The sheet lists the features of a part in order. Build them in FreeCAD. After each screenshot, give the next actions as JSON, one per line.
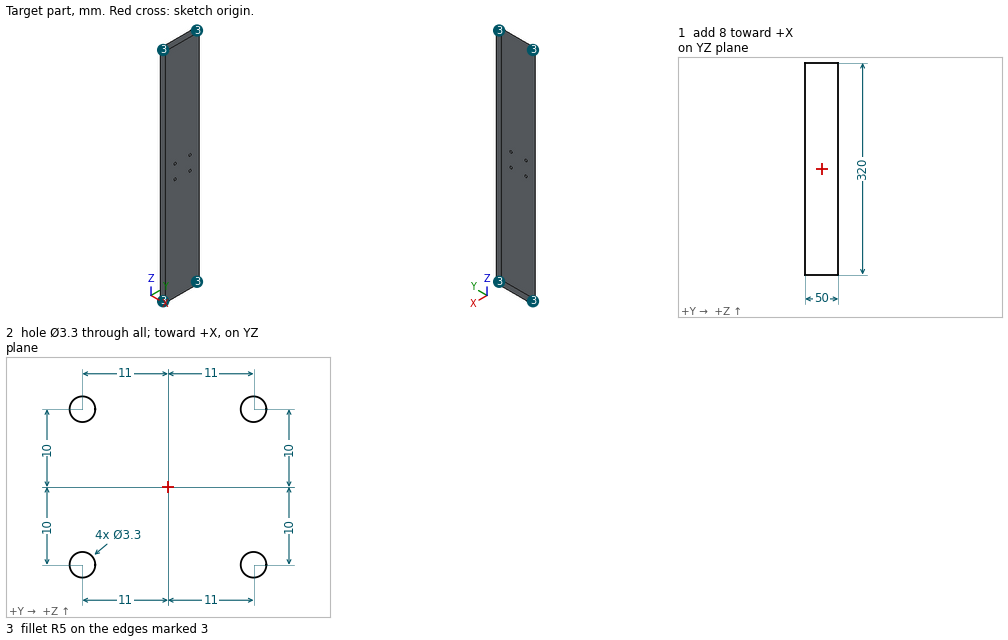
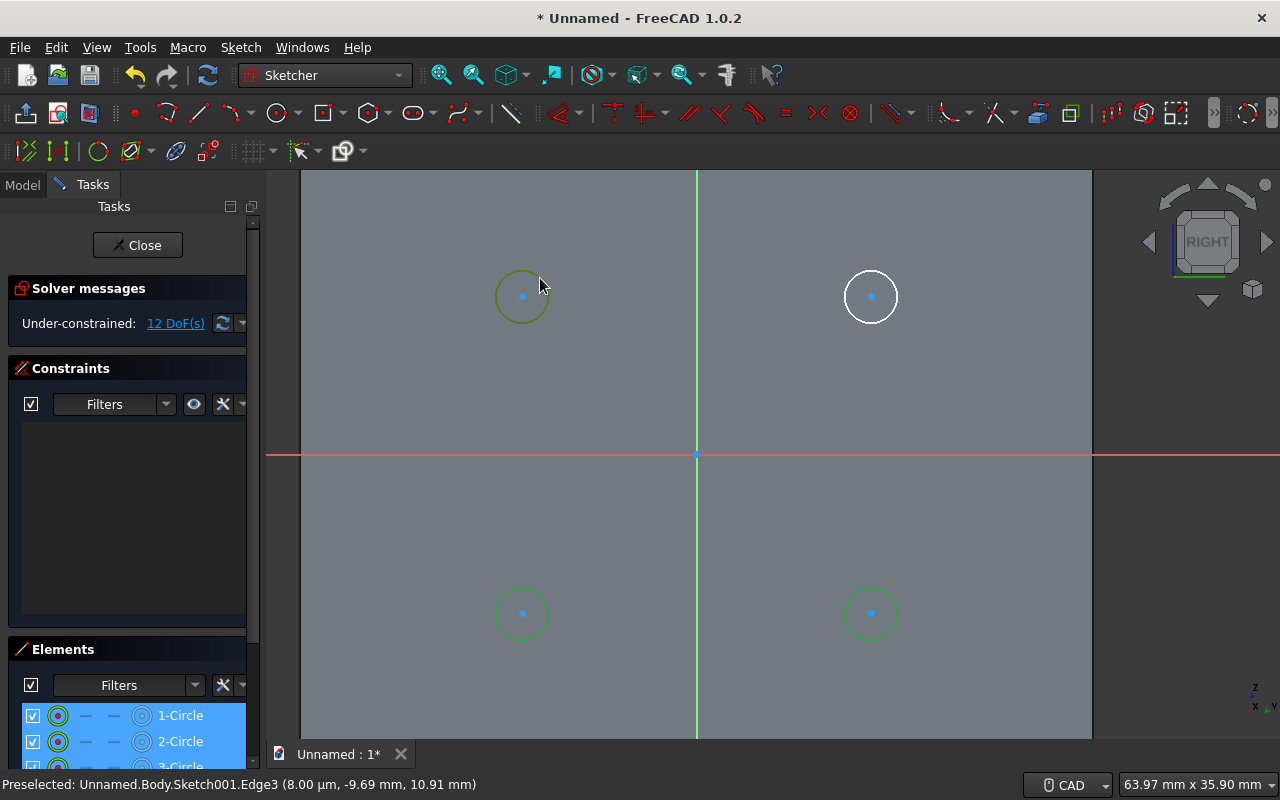
{"action": "left_click", "coordinate": [889, 278]}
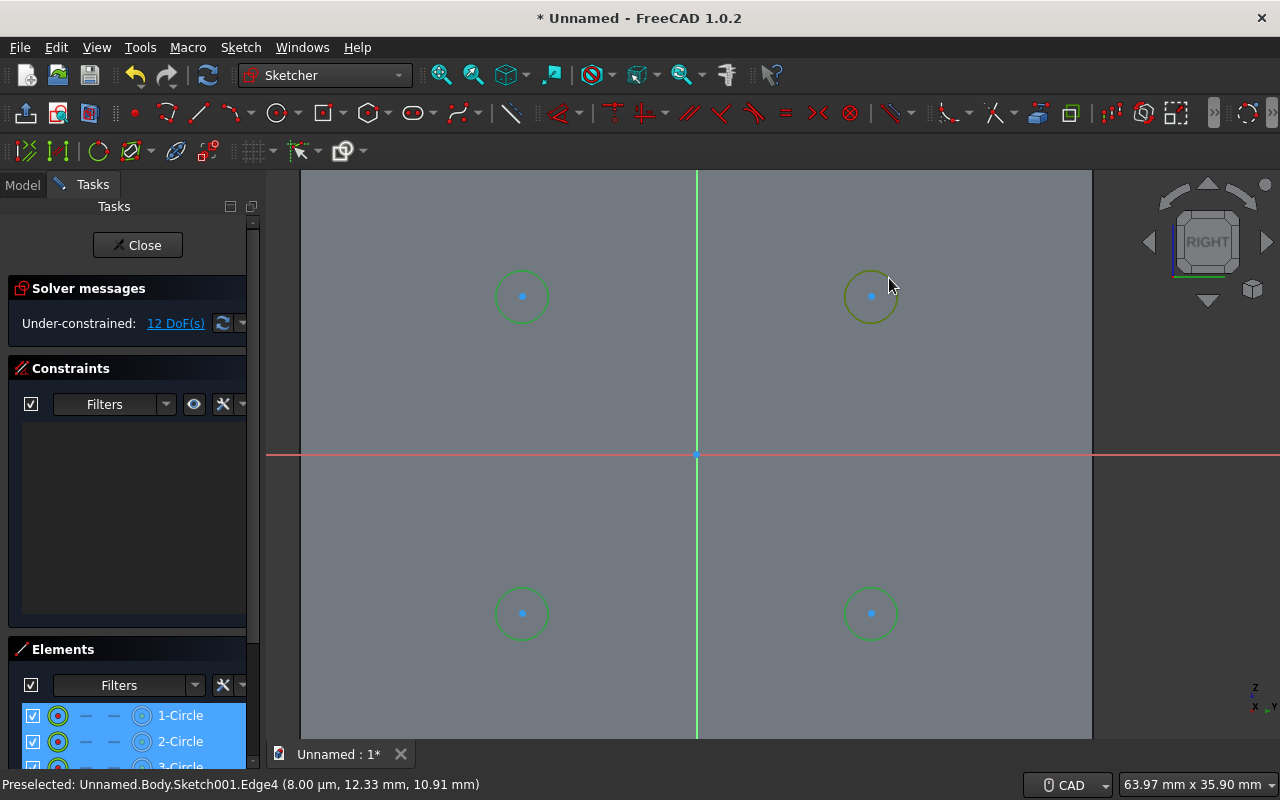
{"action": "left_click", "coordinate": [786, 114]}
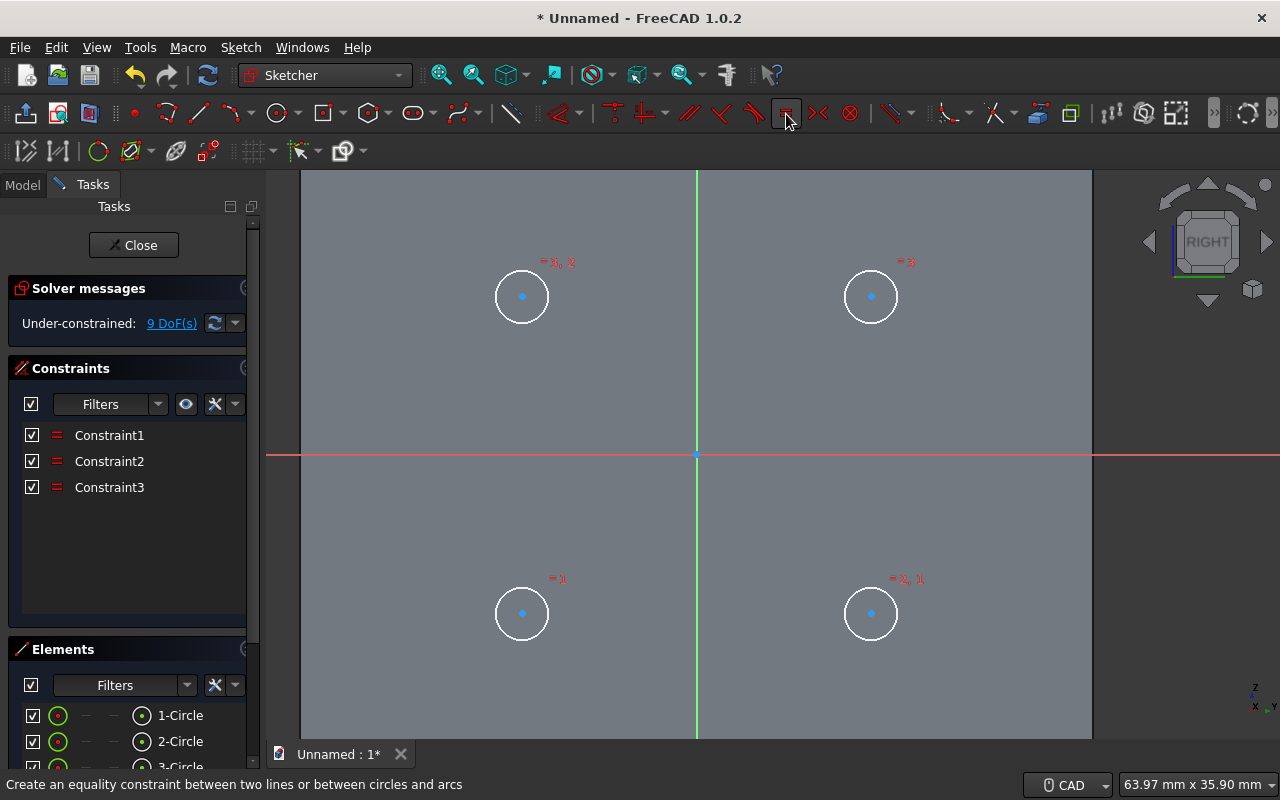
{"action": "key", "text": "d"}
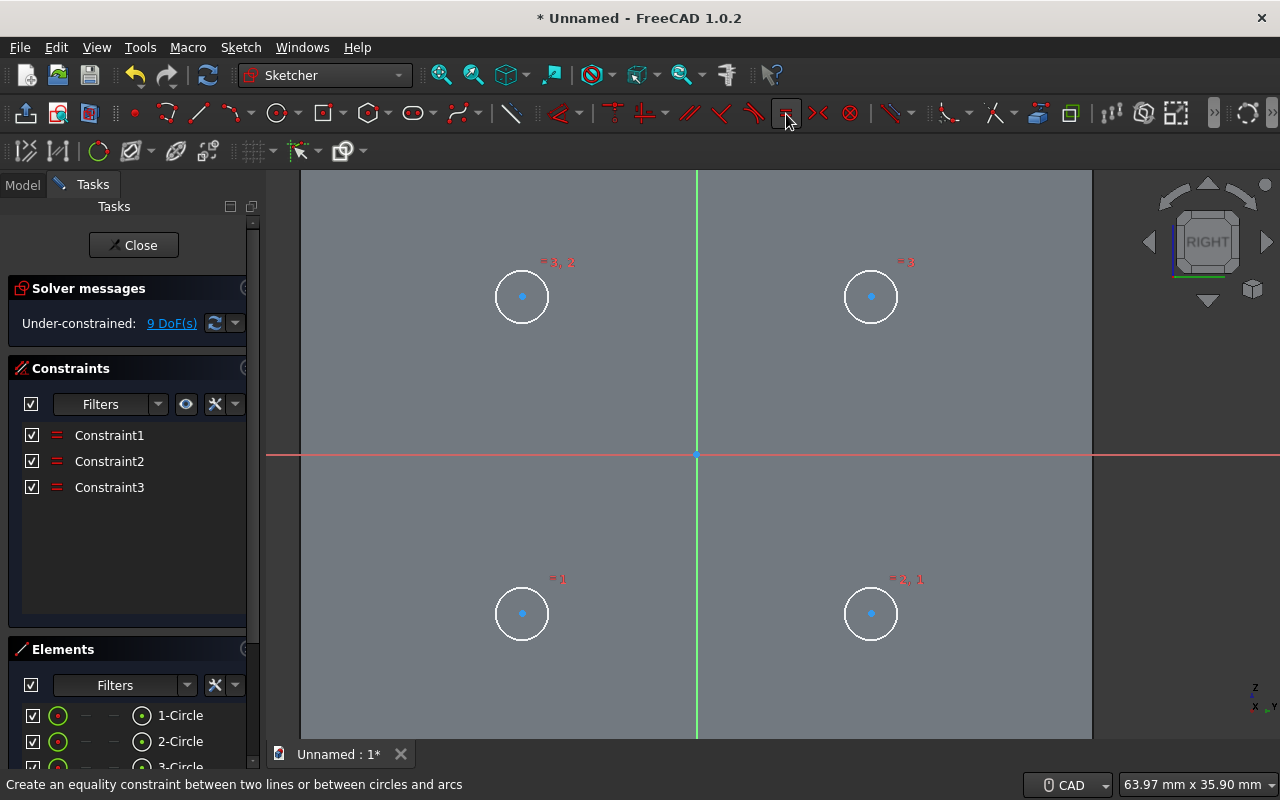
{"action": "left_click", "coordinate": [540, 595]}
{"action": "left_click", "coordinate": [562, 572]}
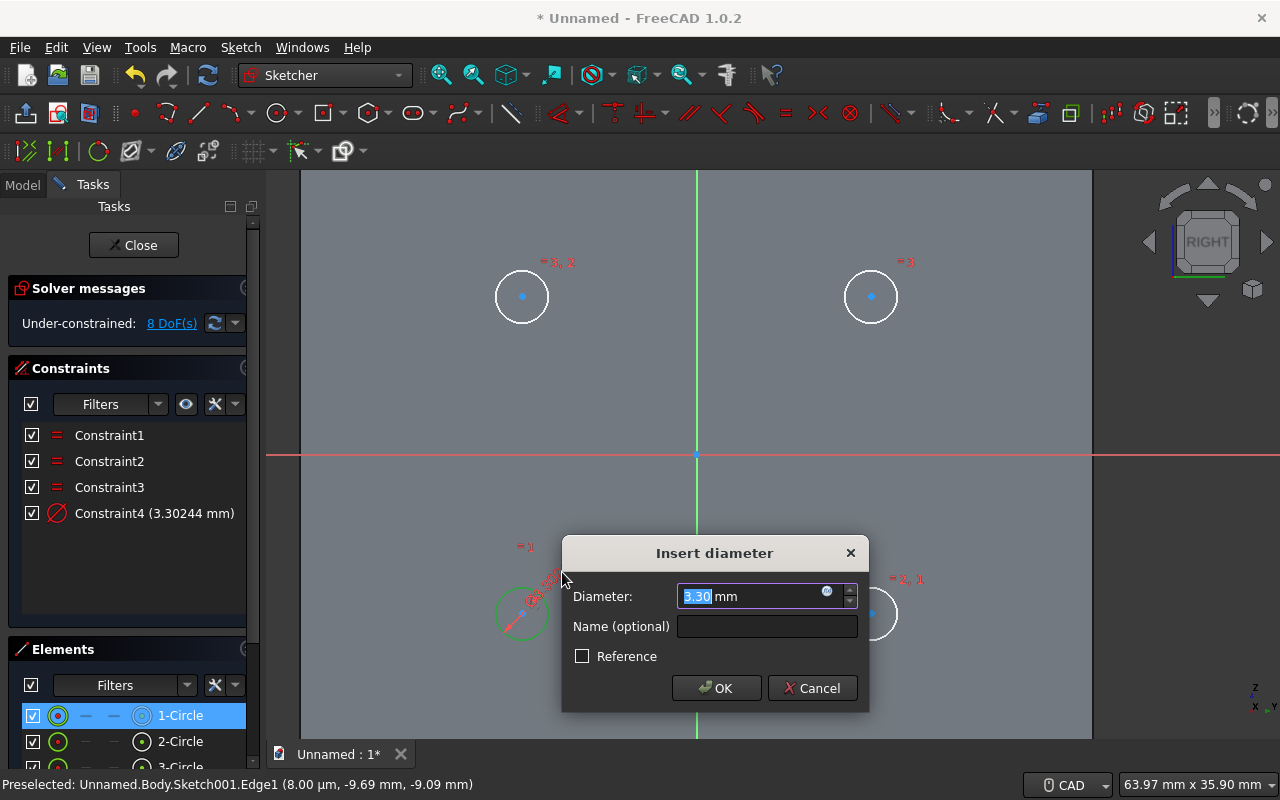
{"action": "type", "text": "3.3"}
{"action": "key", "text": "Return"}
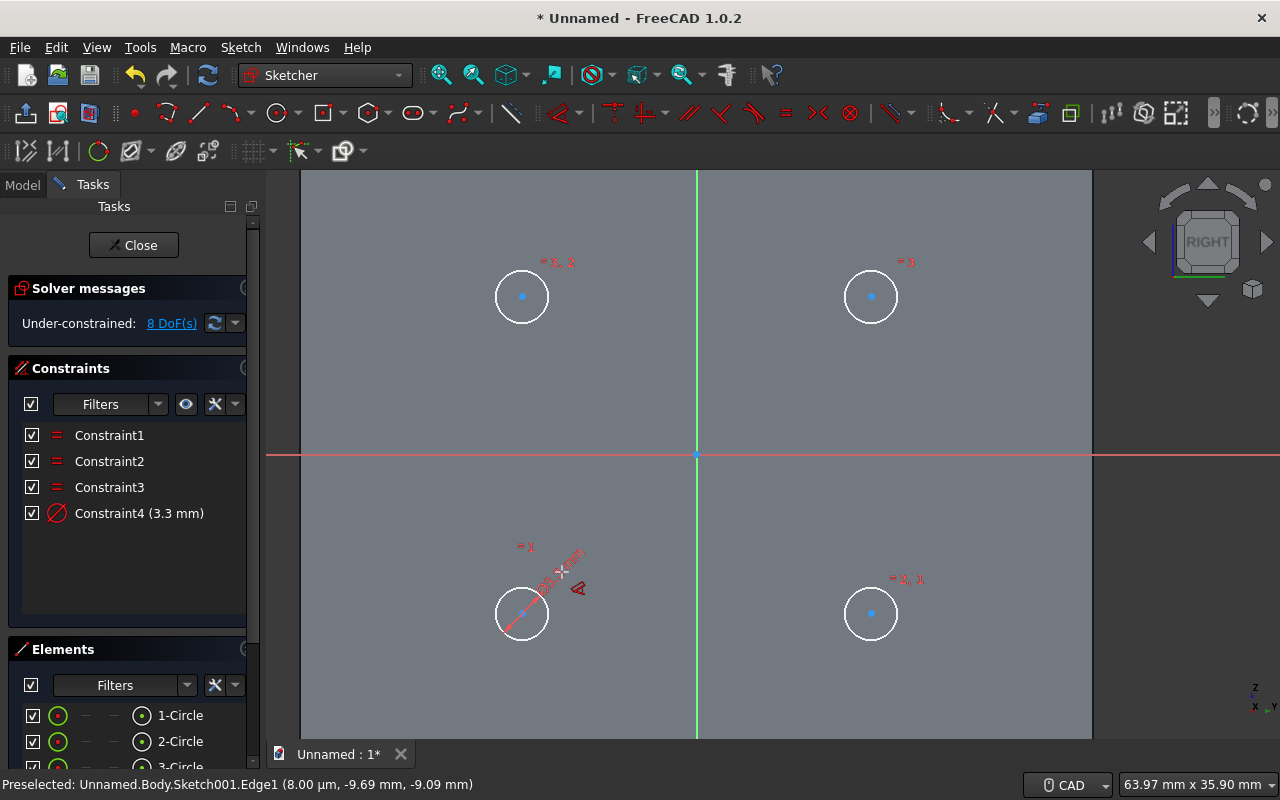
{"action": "left_click", "coordinate": [522, 614]}
{"action": "left_click", "coordinate": [609, 648]}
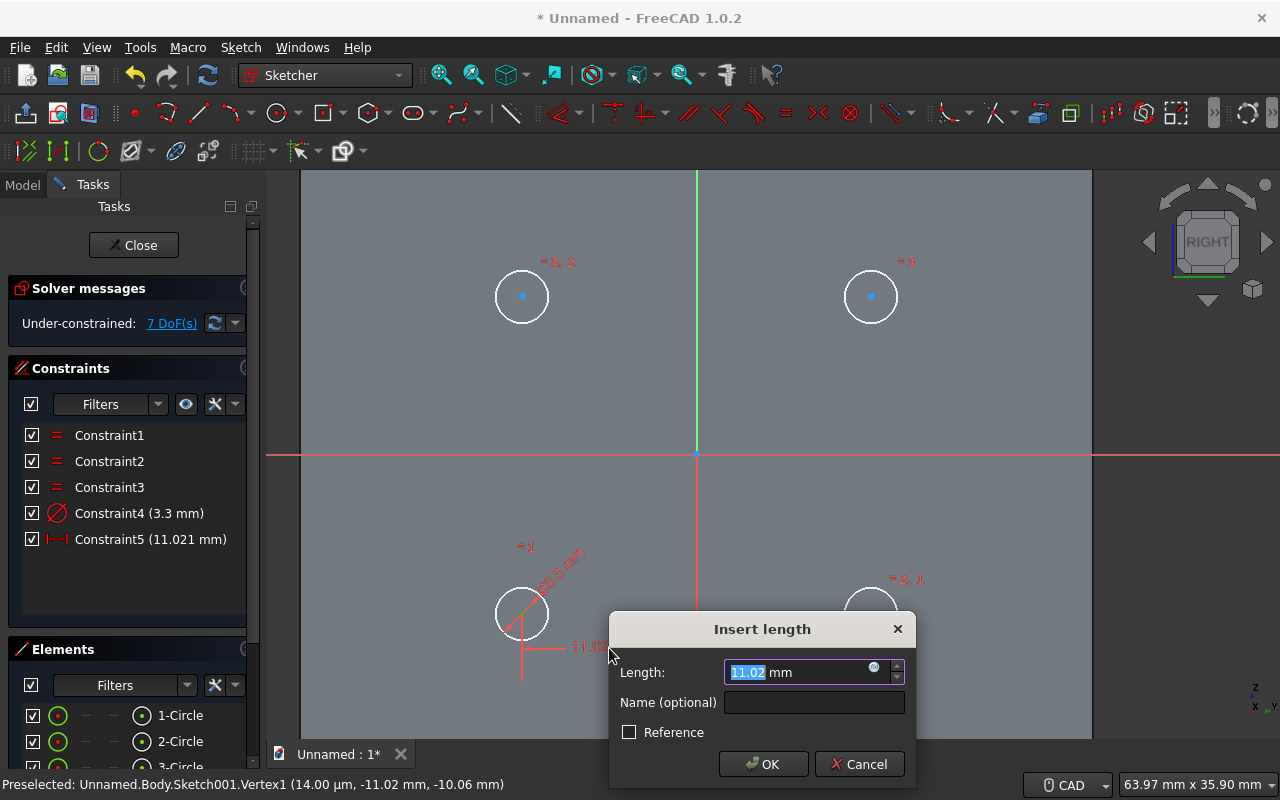
{"action": "type", "text": "11"}
{"action": "key", "text": "Return"}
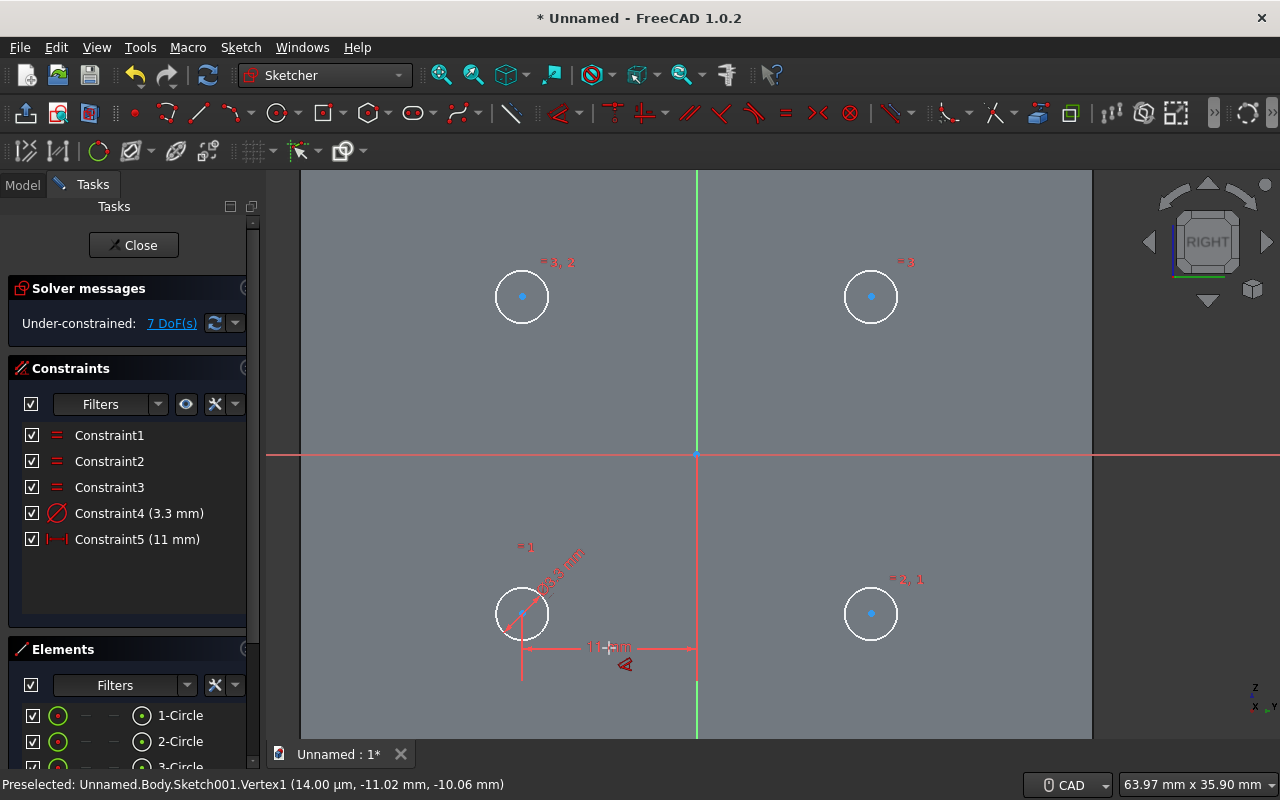
{"action": "left_click", "coordinate": [522, 614]}
{"action": "left_click", "coordinate": [488, 534]}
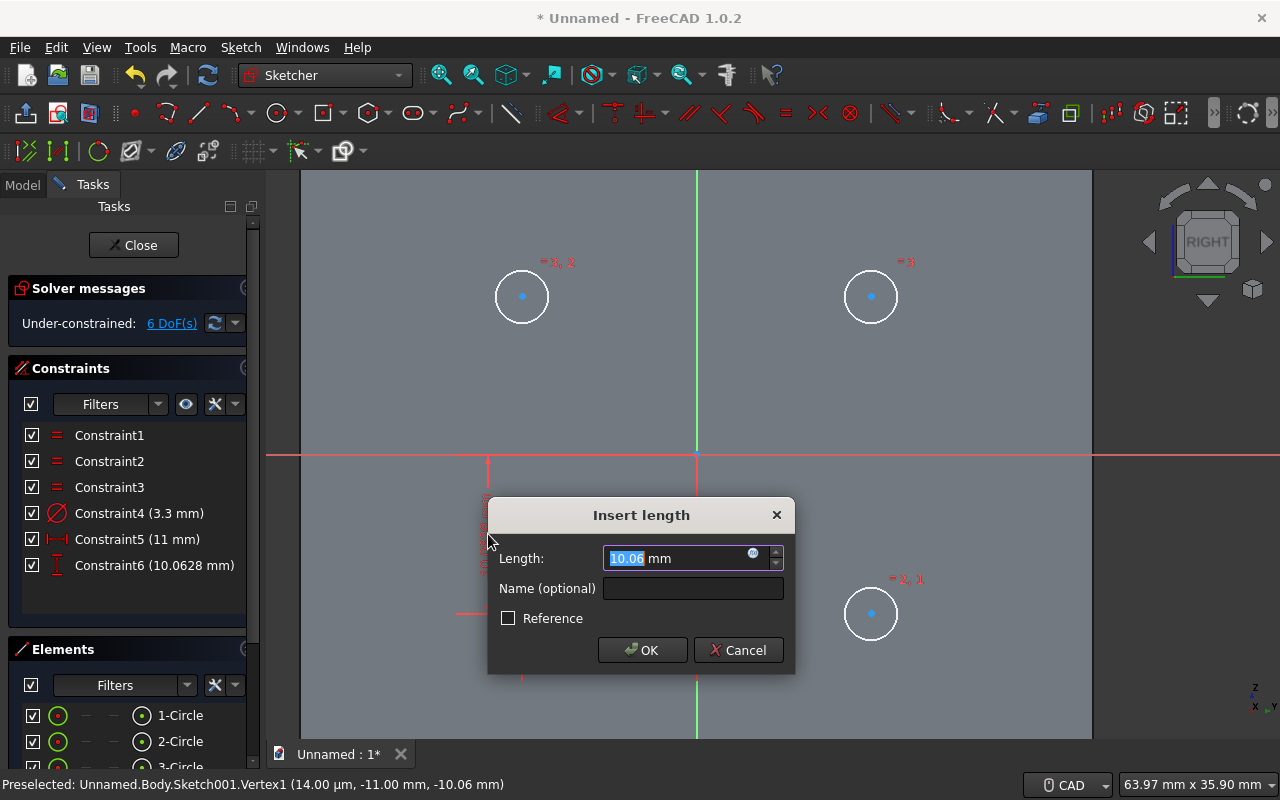
{"action": "type", "text": "10"}
{"action": "key", "text": "Return"}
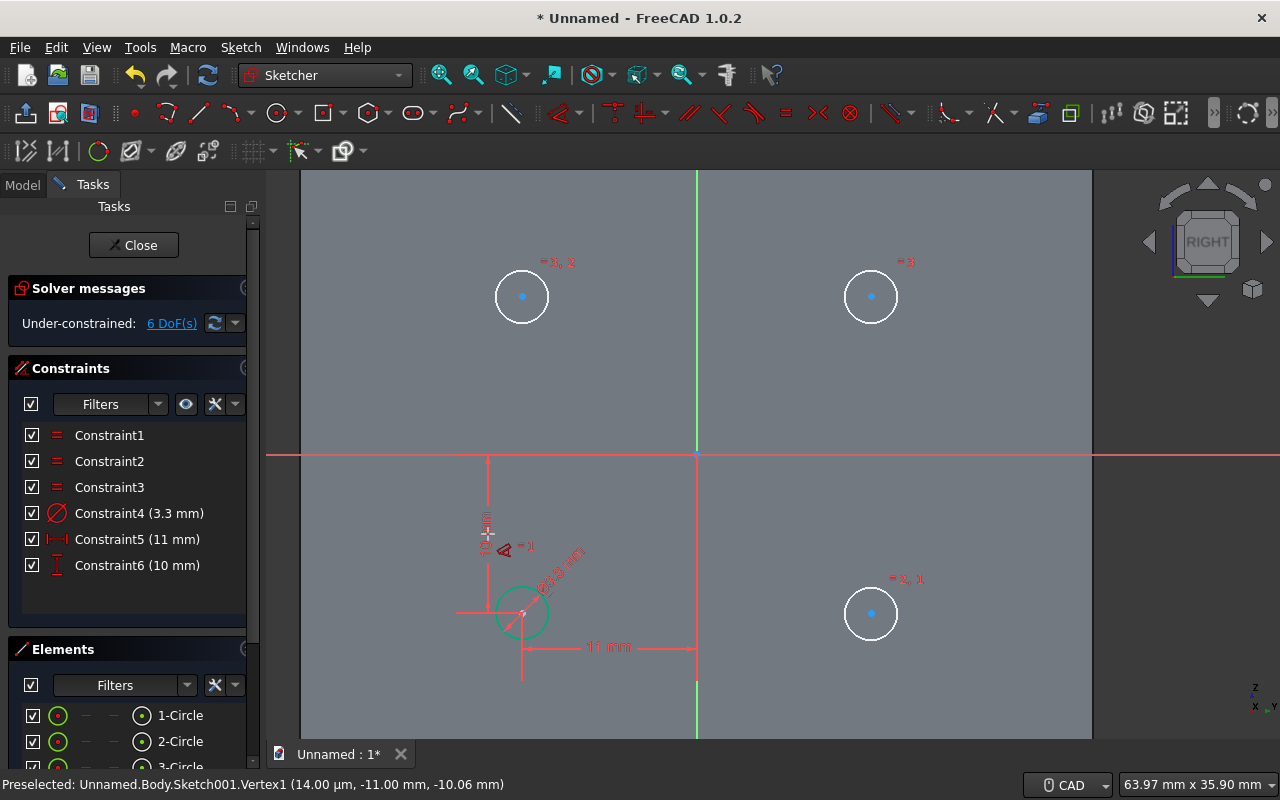
{"action": "left_click", "coordinate": [871, 614]}
{"action": "left_click", "coordinate": [784, 648]}